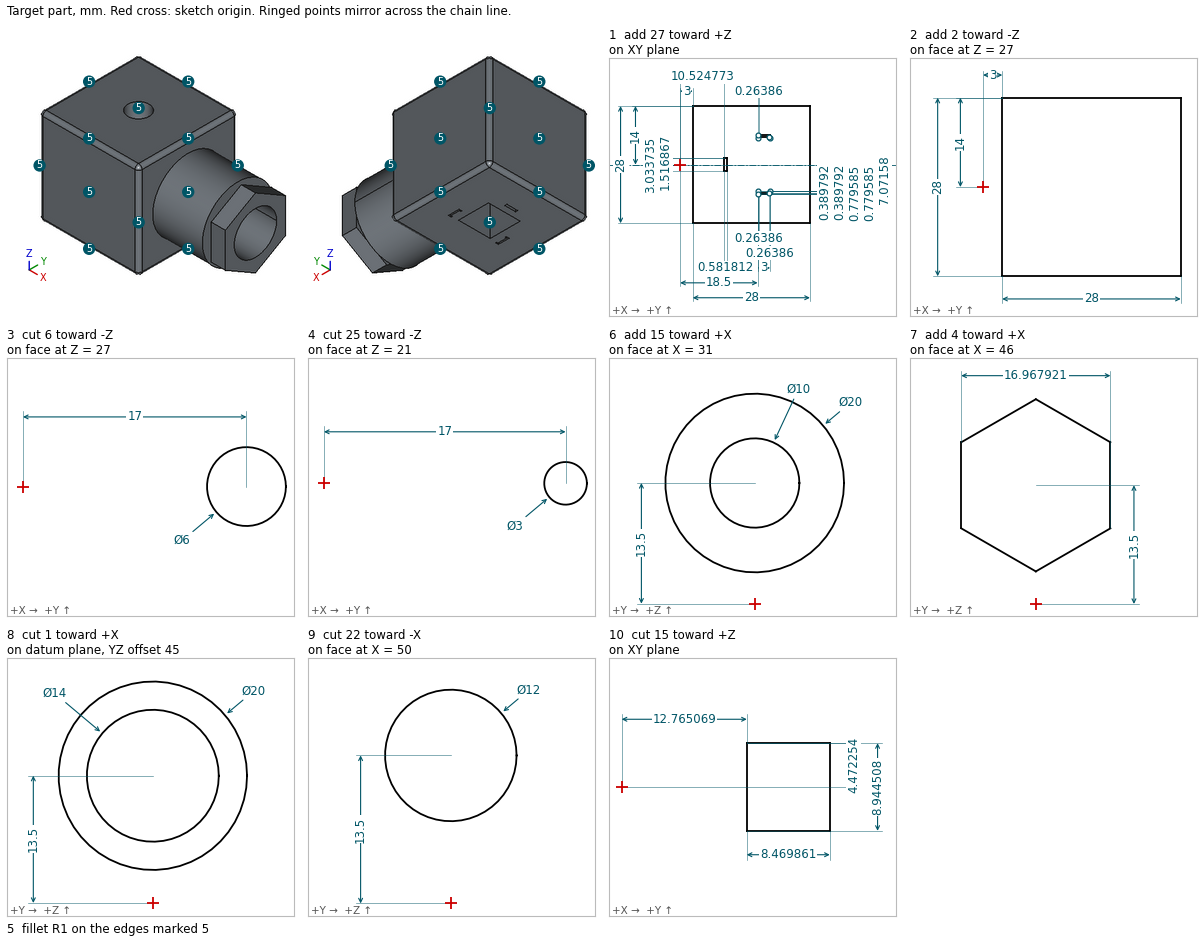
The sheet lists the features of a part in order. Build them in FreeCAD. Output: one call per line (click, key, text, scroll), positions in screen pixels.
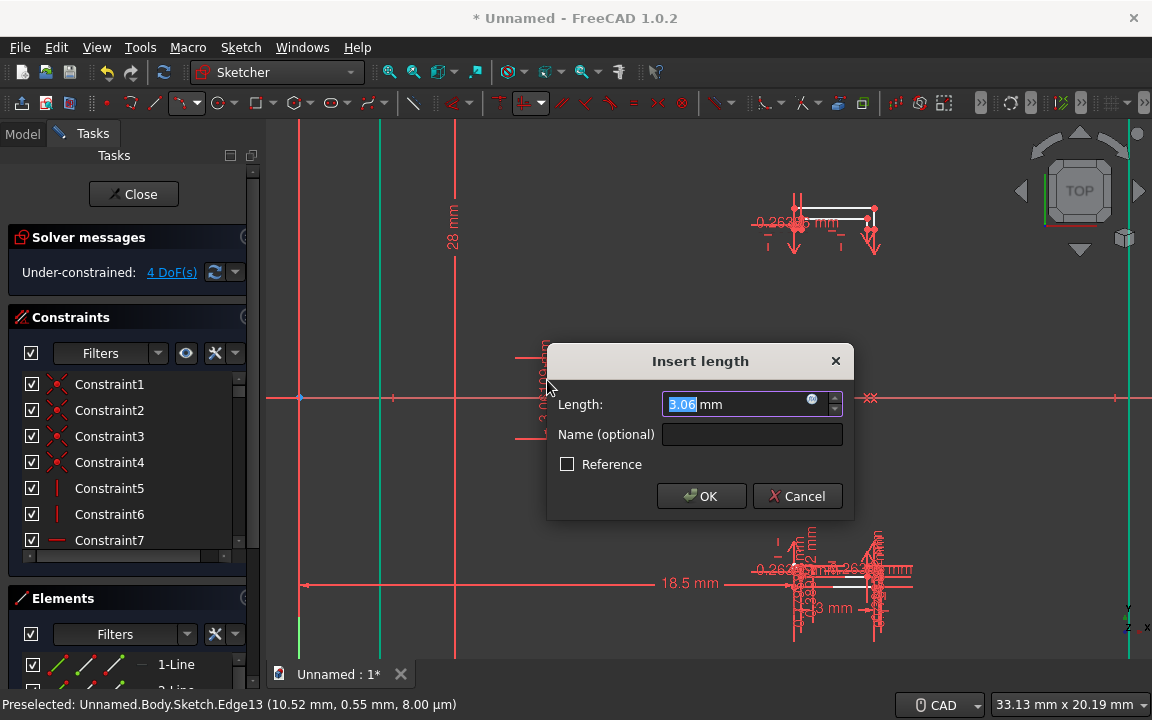
text(3.033735)
key(Return)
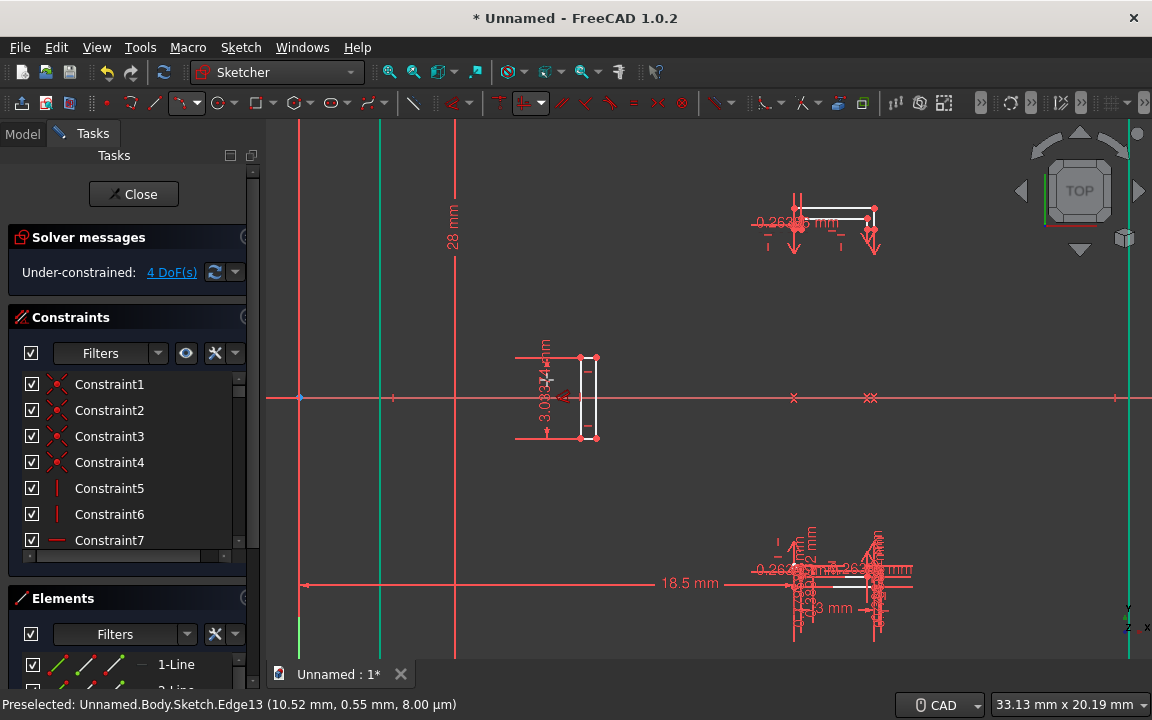
scroll(589, 439, up, 5)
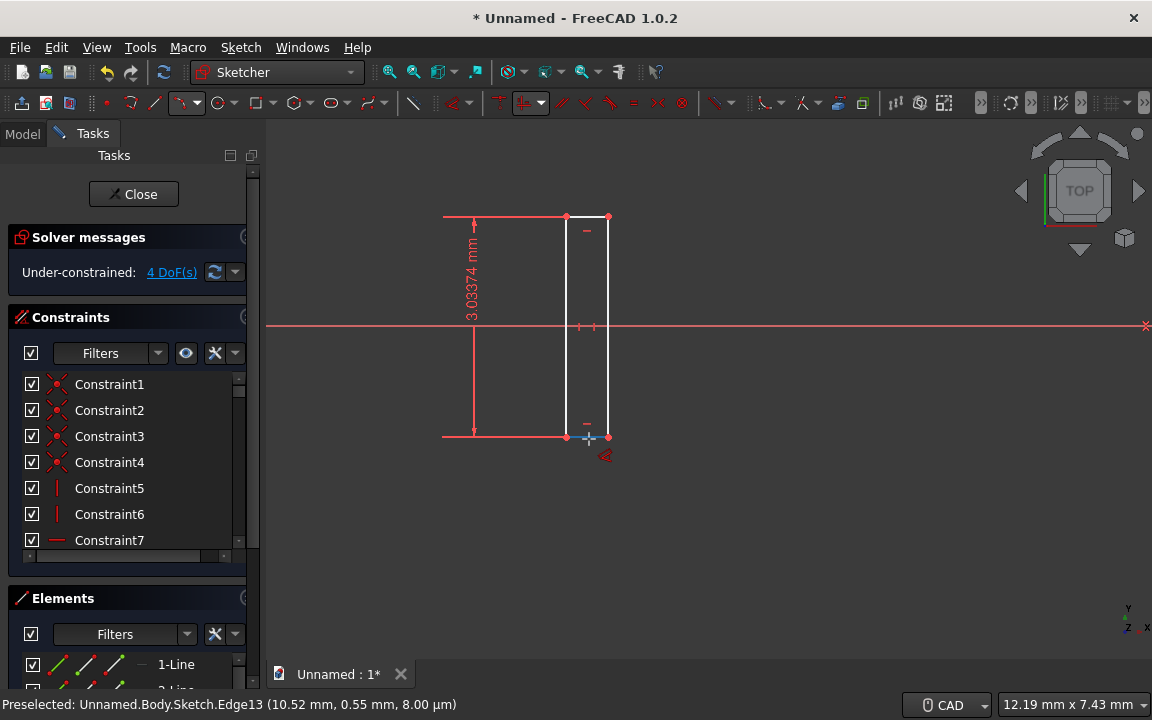
click(587, 437)
click(587, 471)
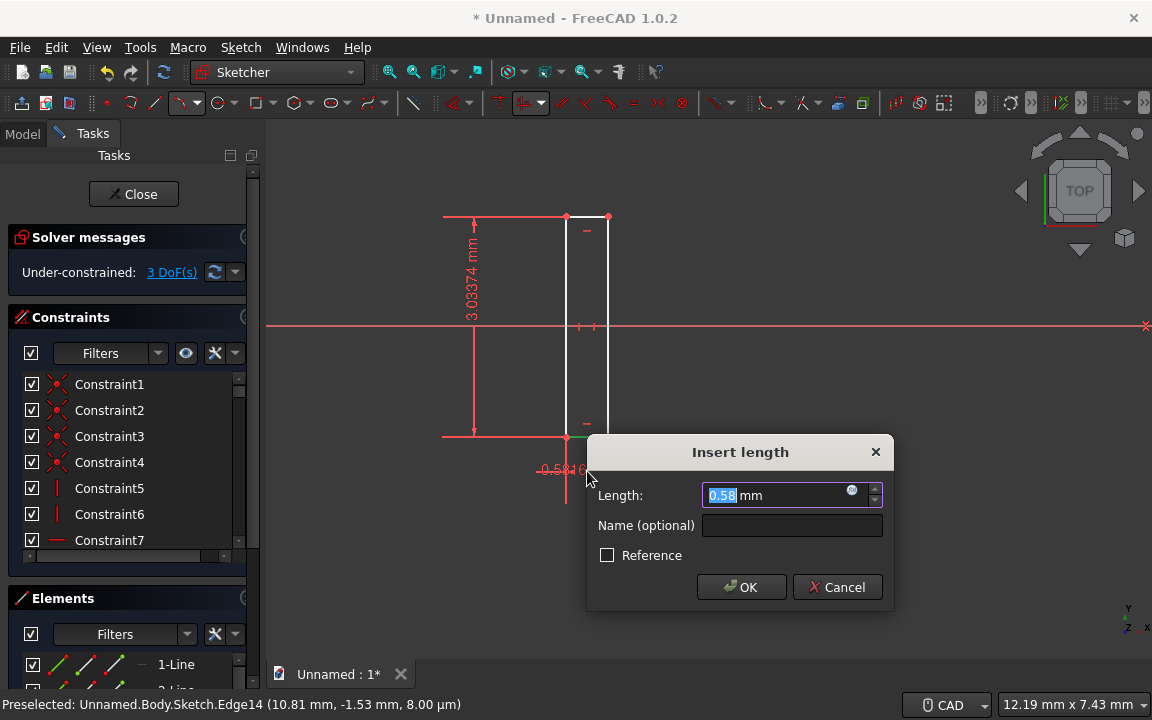
text(0.581812)
key(Return)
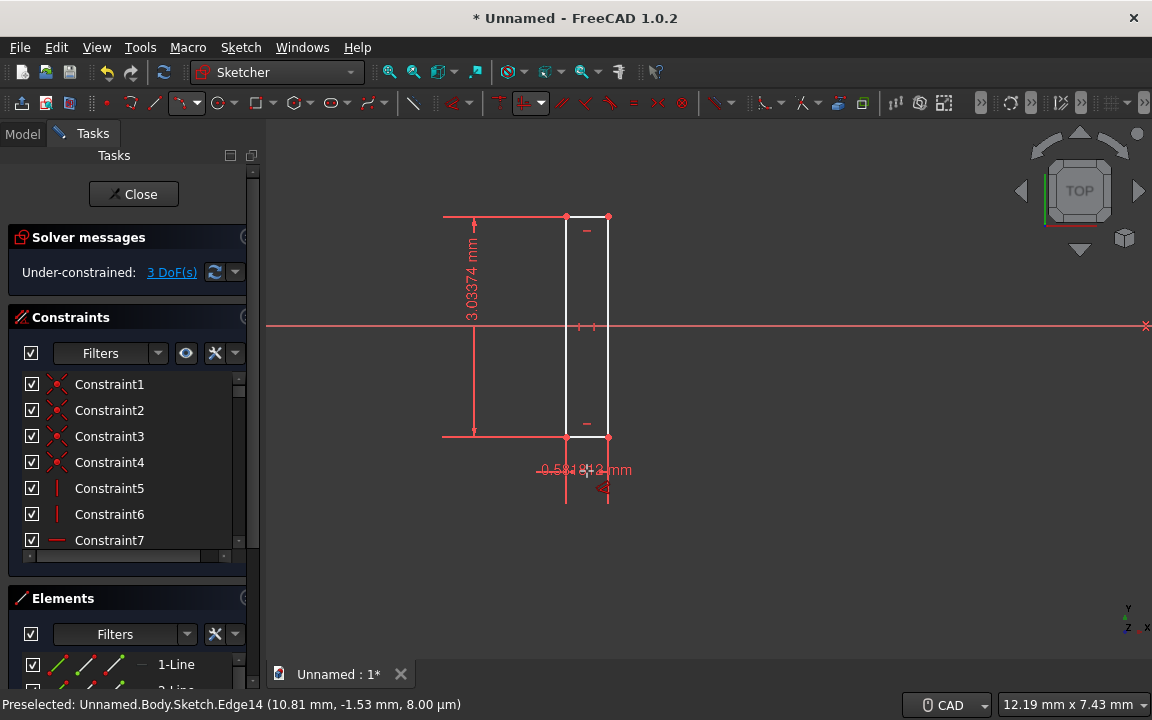
scroll(584, 402, down, 9)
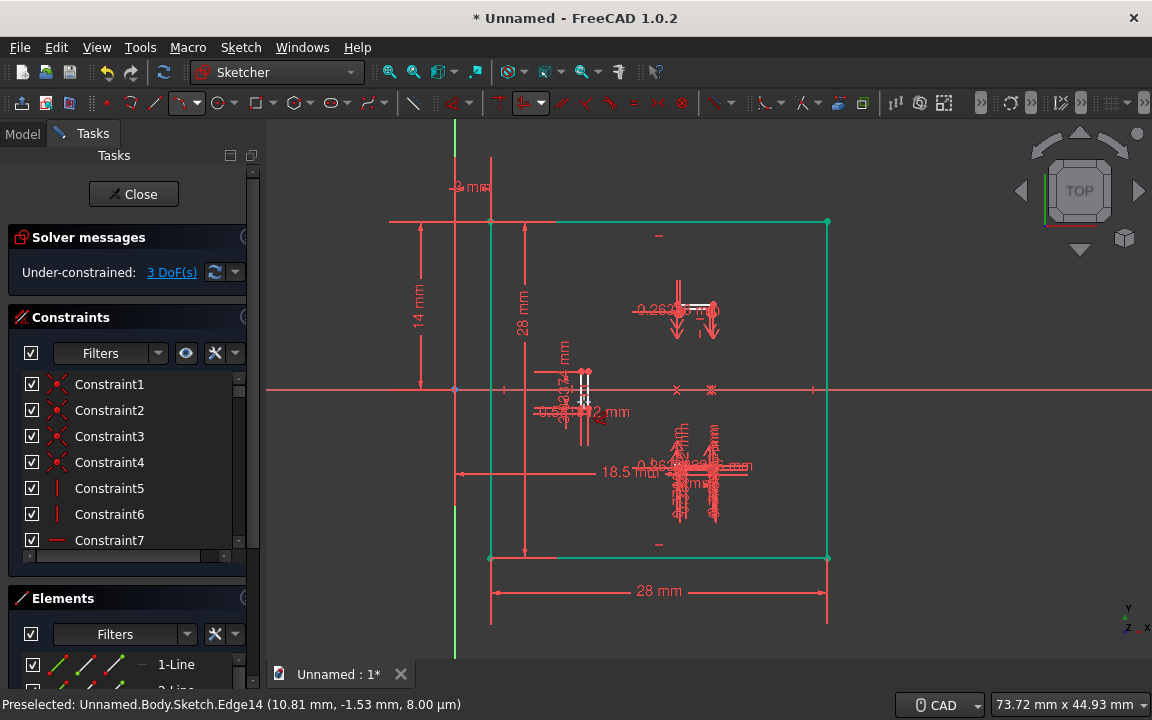
scroll(713, 475, up, 4)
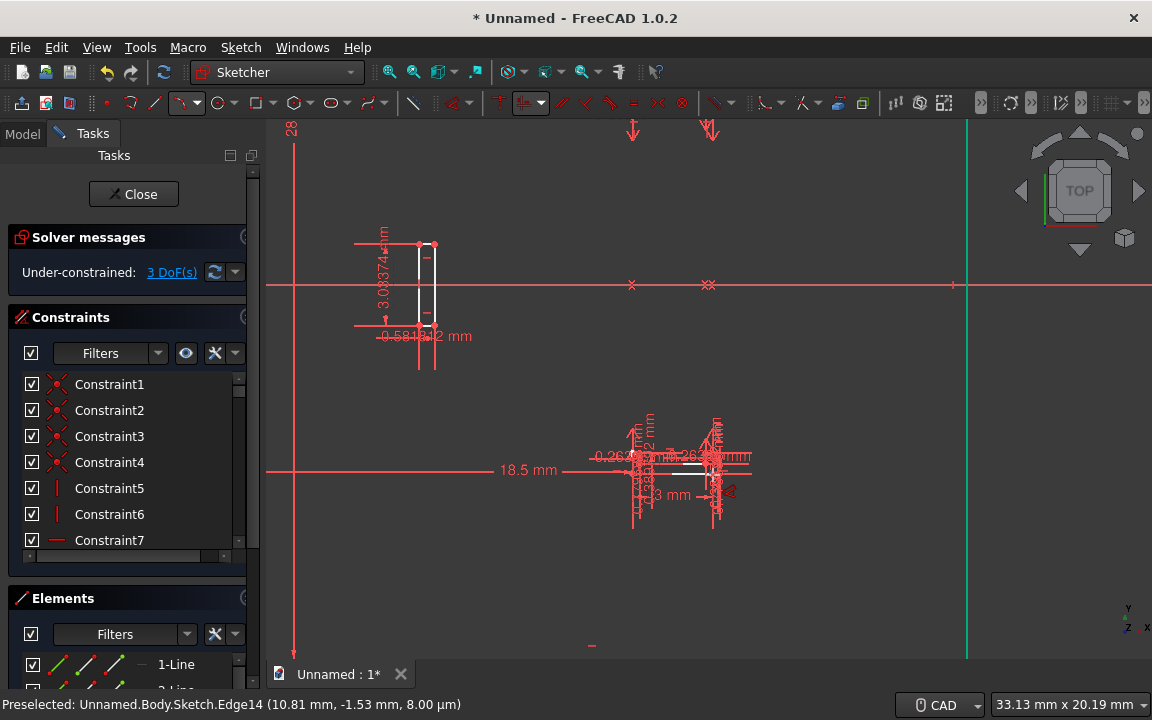
click(713, 474)
click(747, 379)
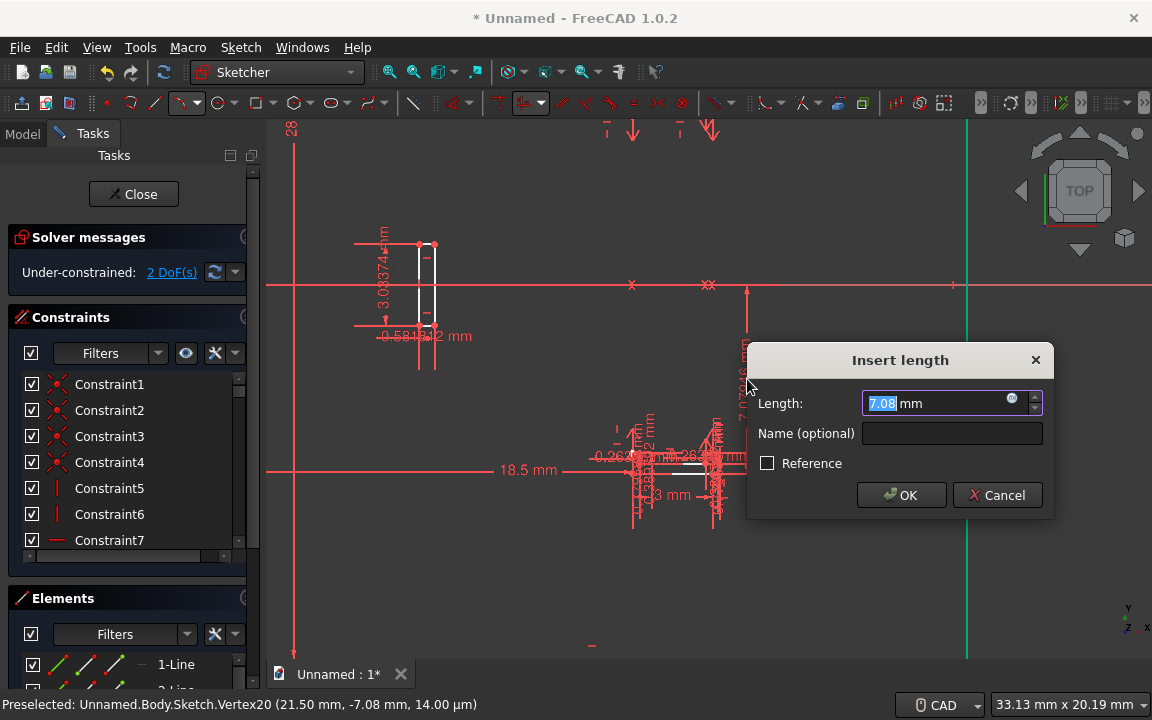
text(7.07158)
key(Return)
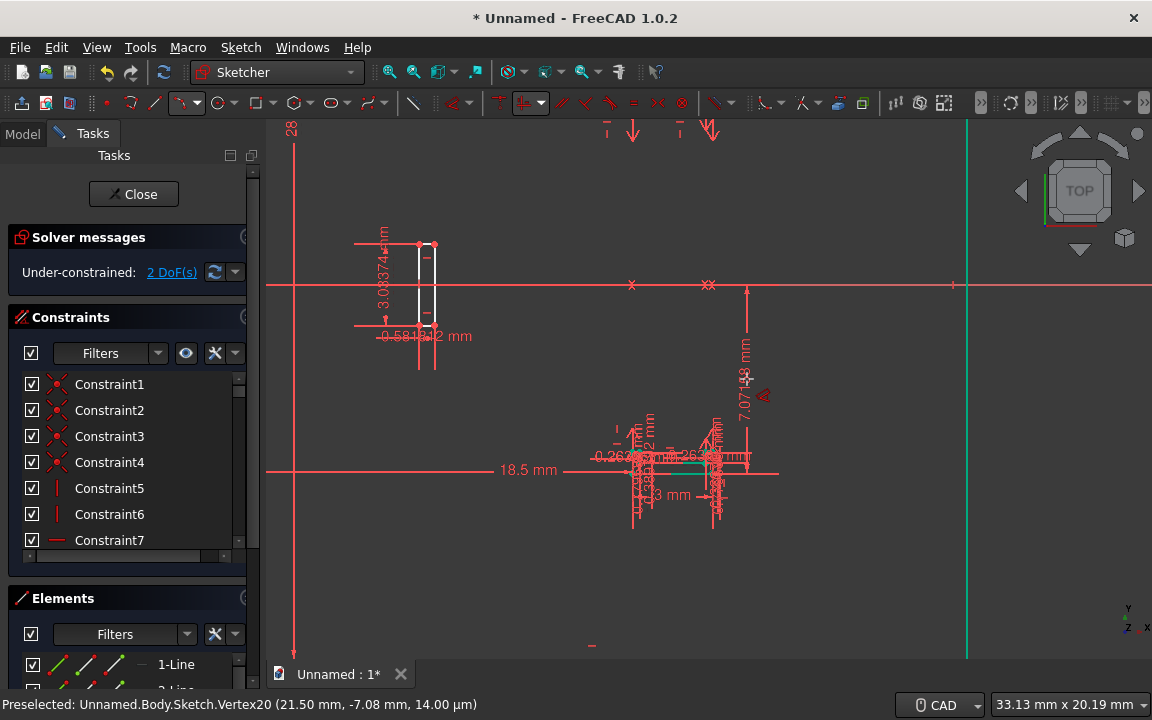
click(419, 244)
click(477, 265)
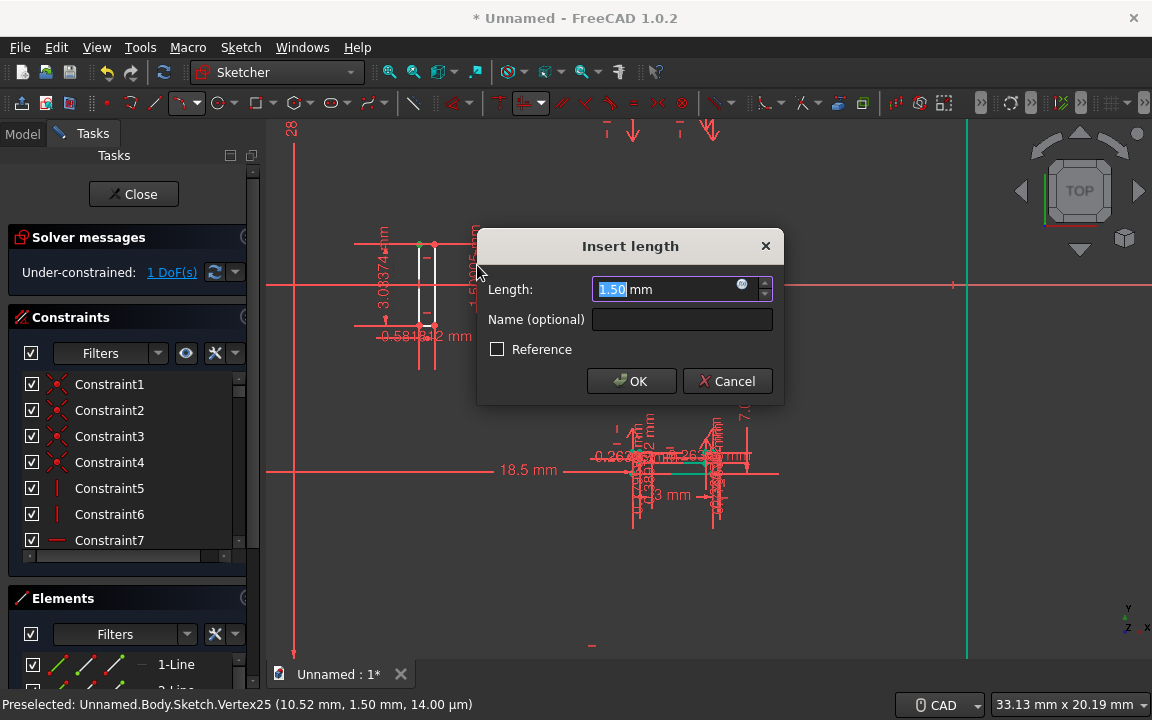
text(1.516867)
key(Return)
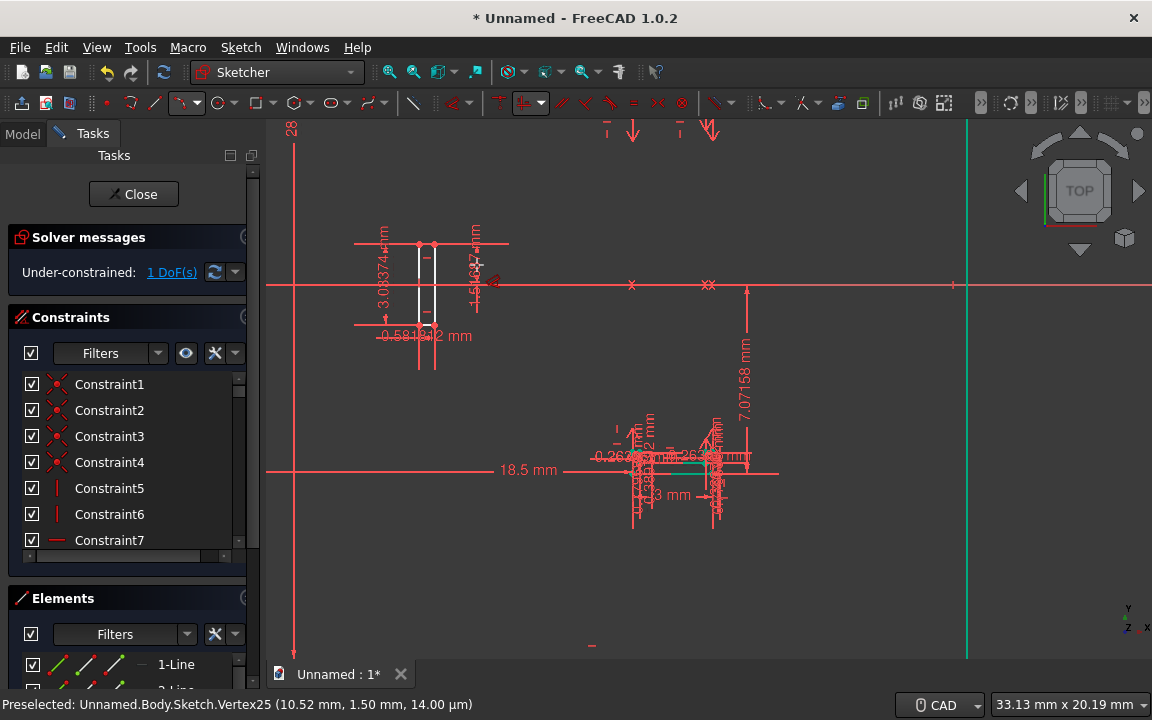
click(419, 244)
click(357, 210)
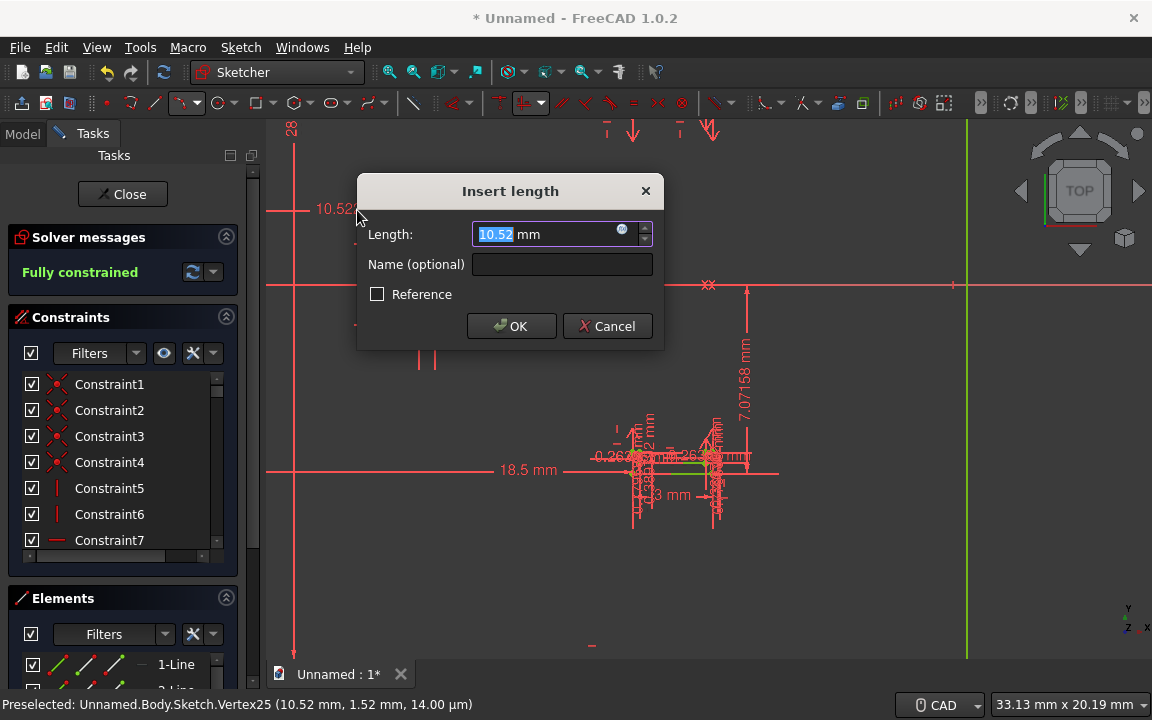
text(10.524773)
key(Return)
key(Escape)